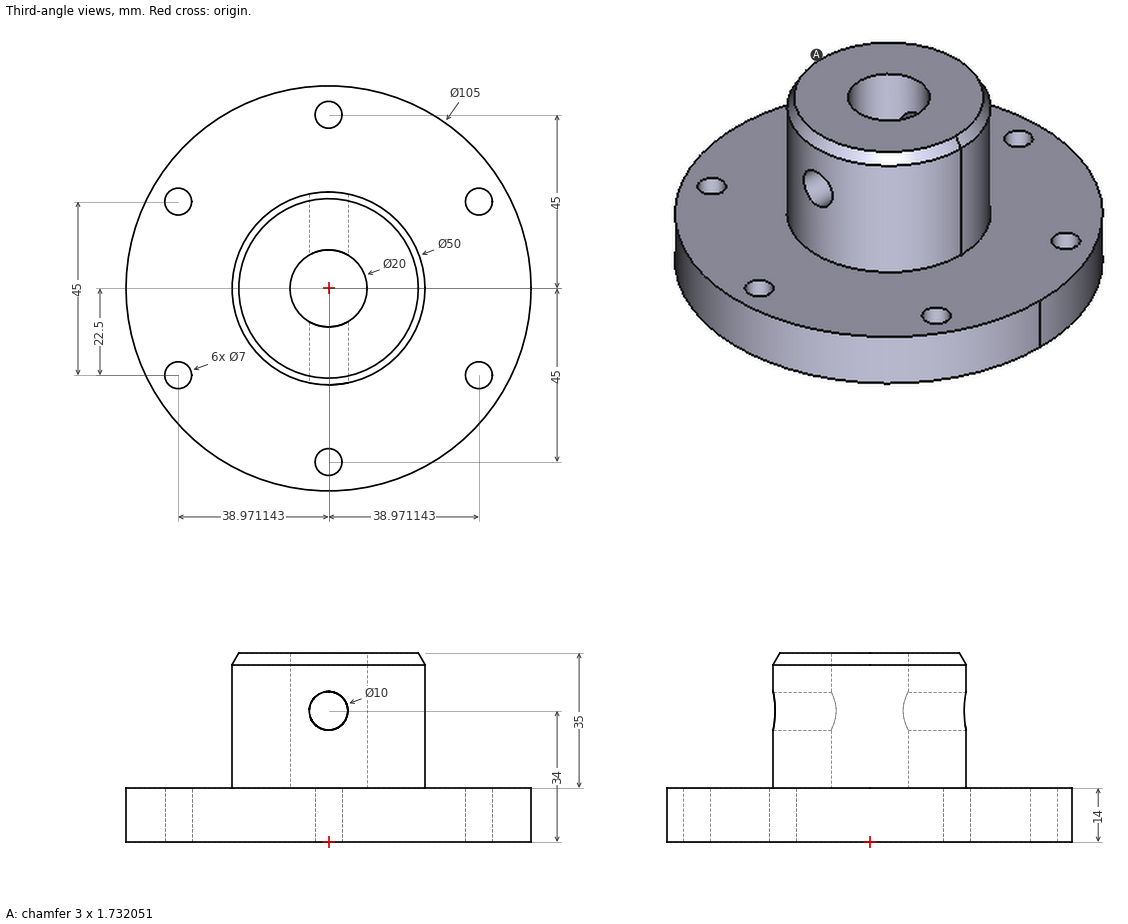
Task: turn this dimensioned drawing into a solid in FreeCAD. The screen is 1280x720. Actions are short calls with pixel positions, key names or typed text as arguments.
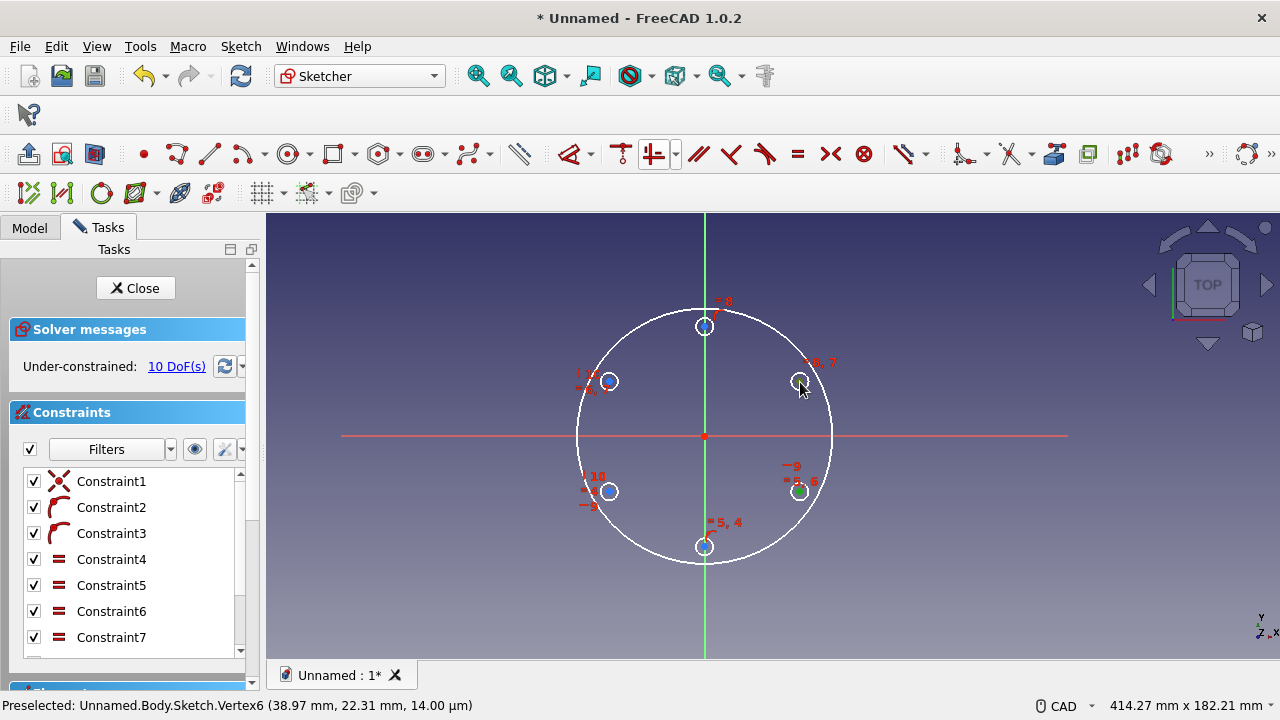
click(676, 154)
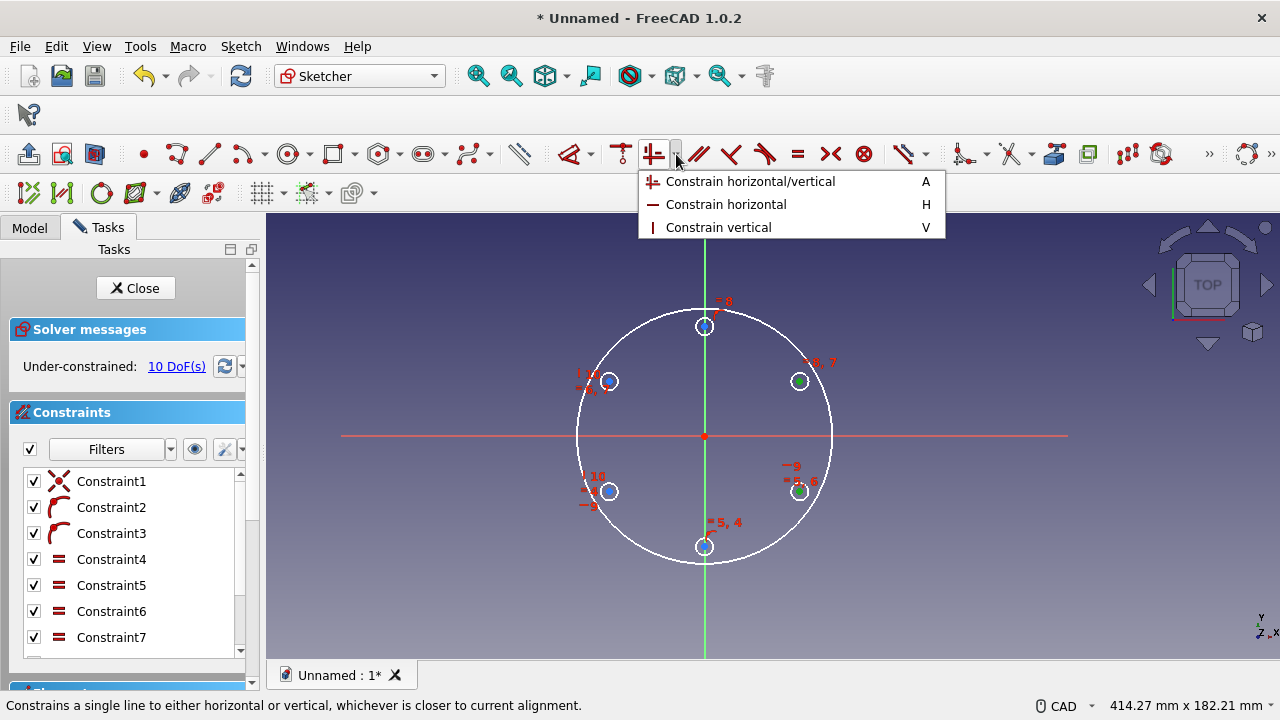
click(792, 228)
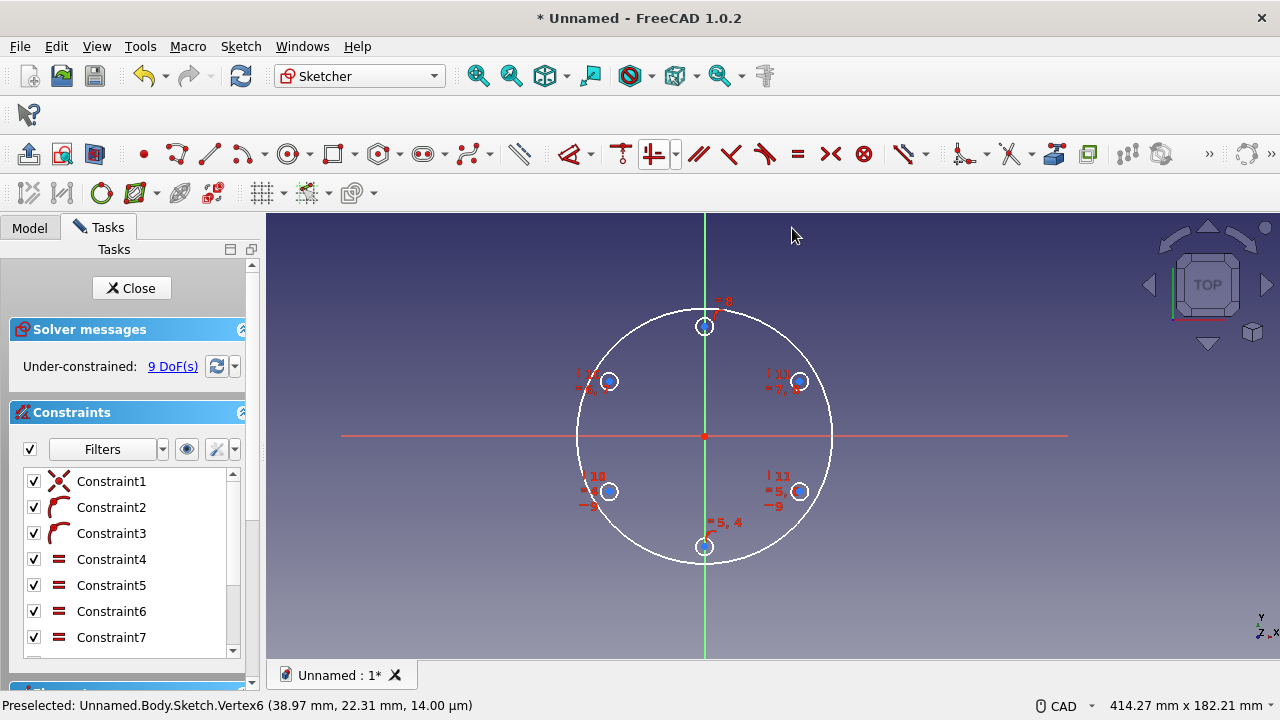
click(611, 384)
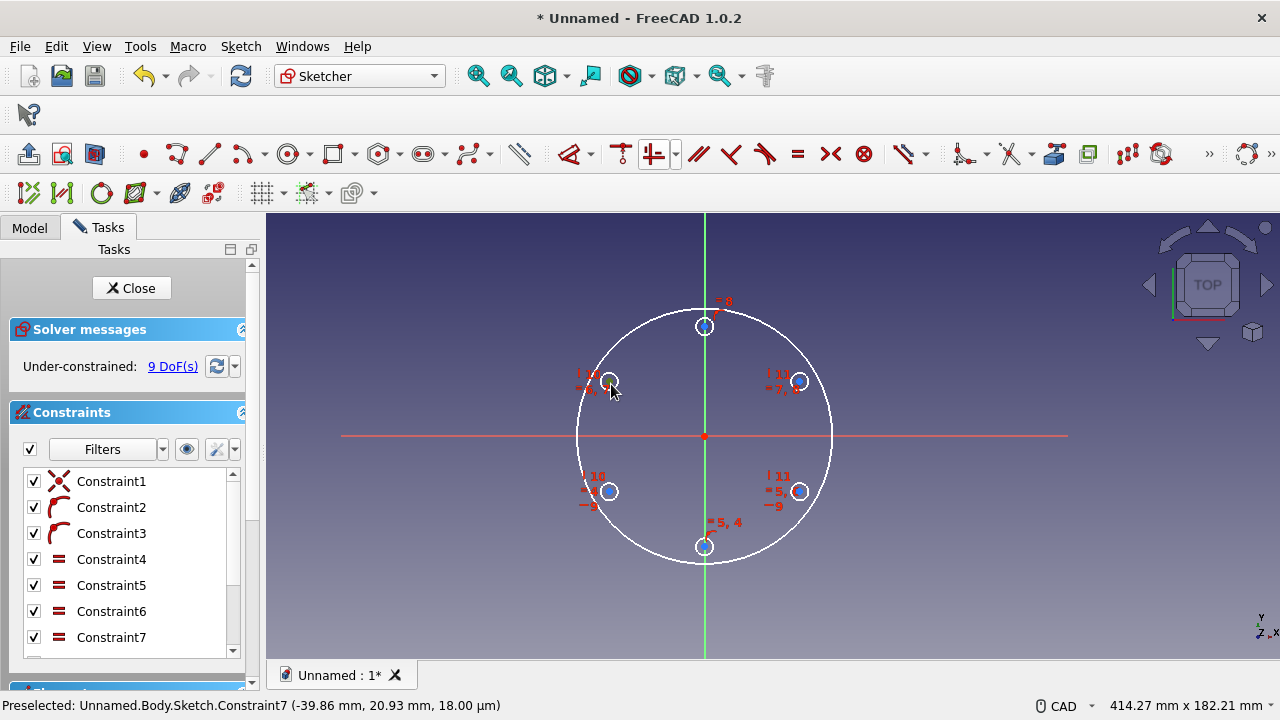
click(802, 384)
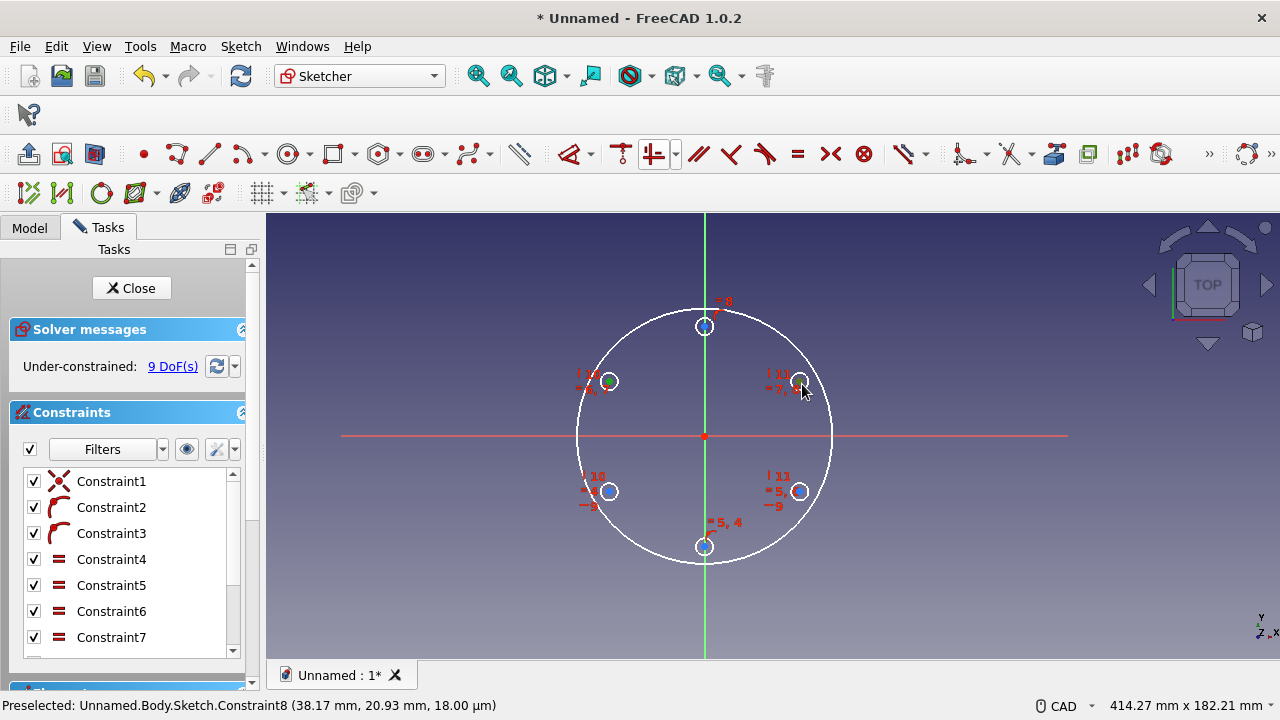
click(676, 154)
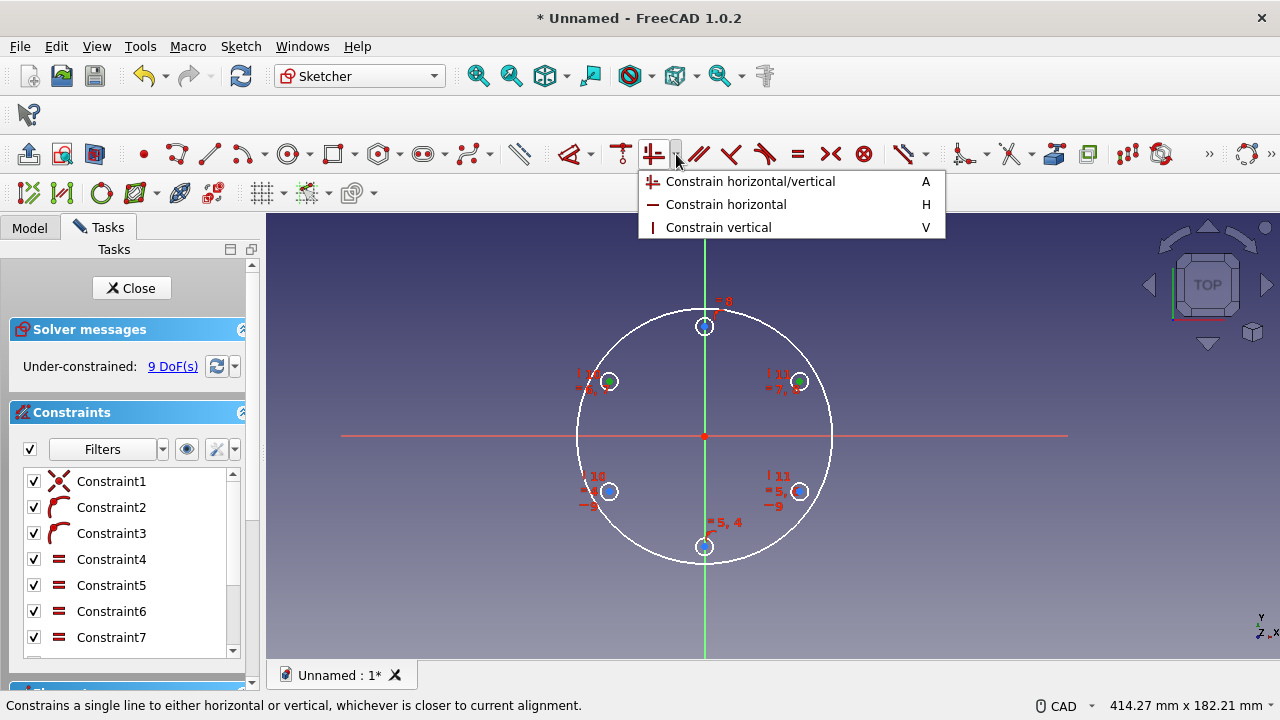
click(792, 204)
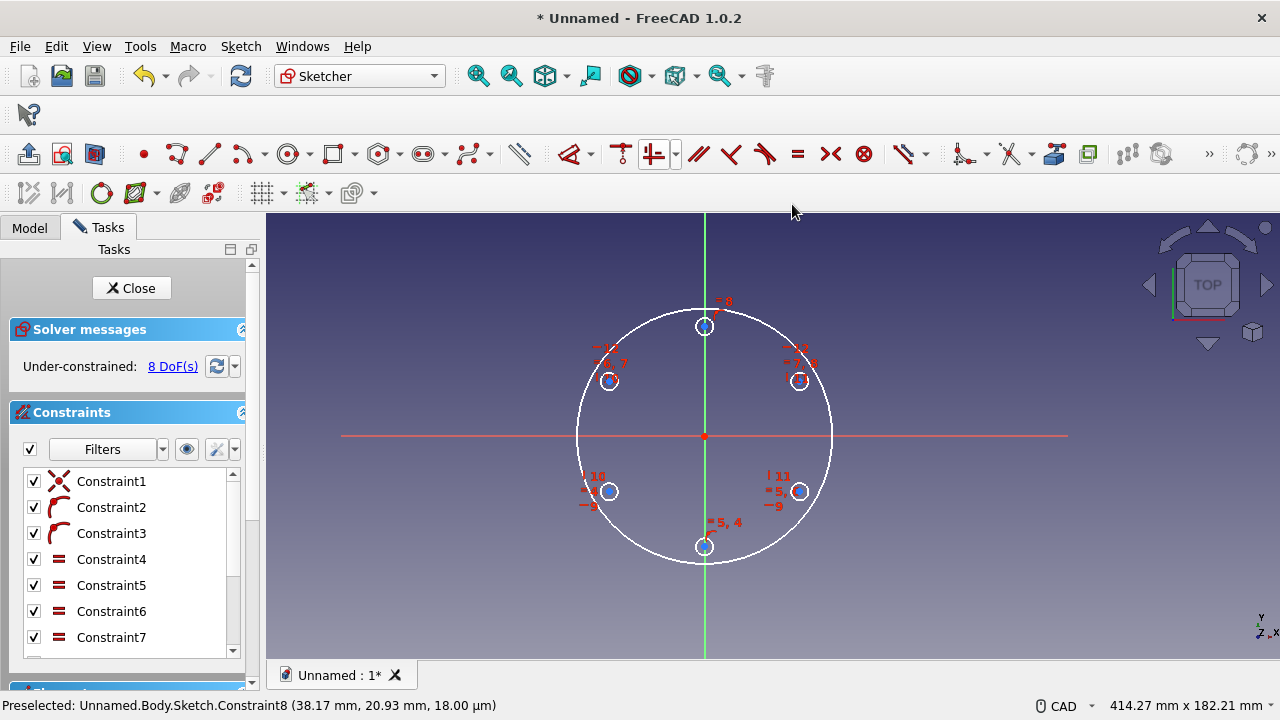
click(568, 154)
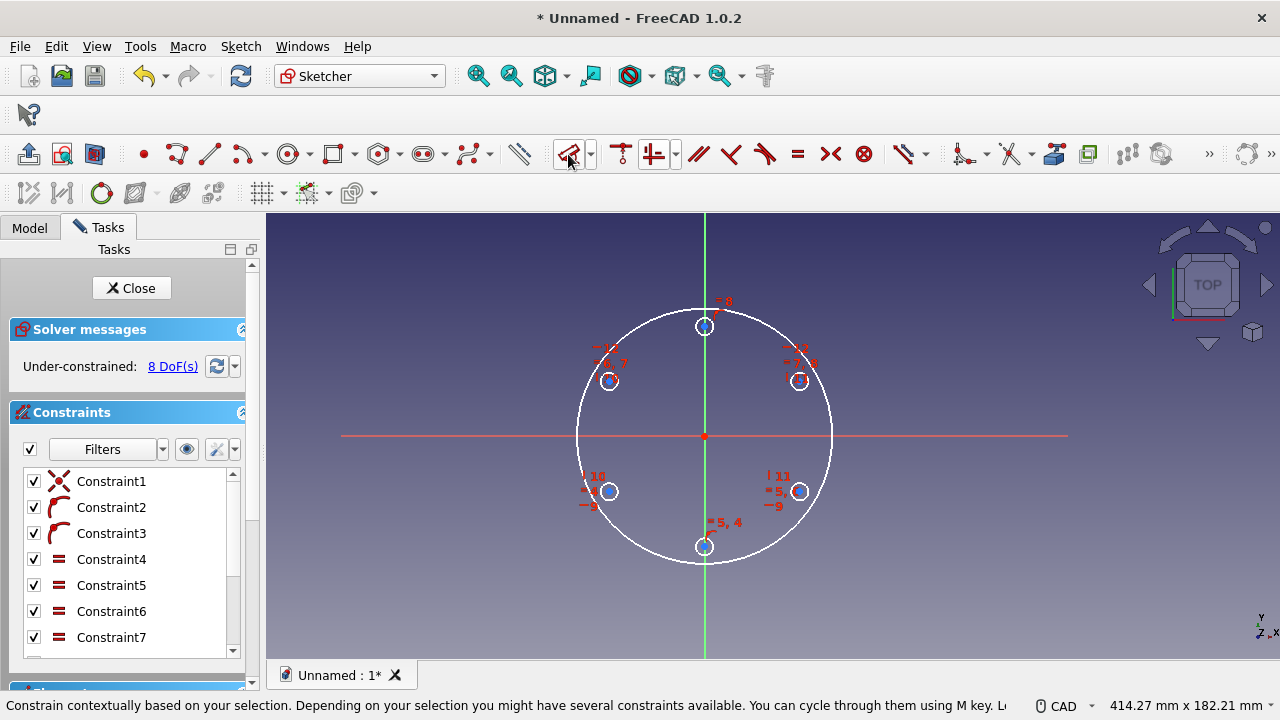
click(795, 346)
click(818, 323)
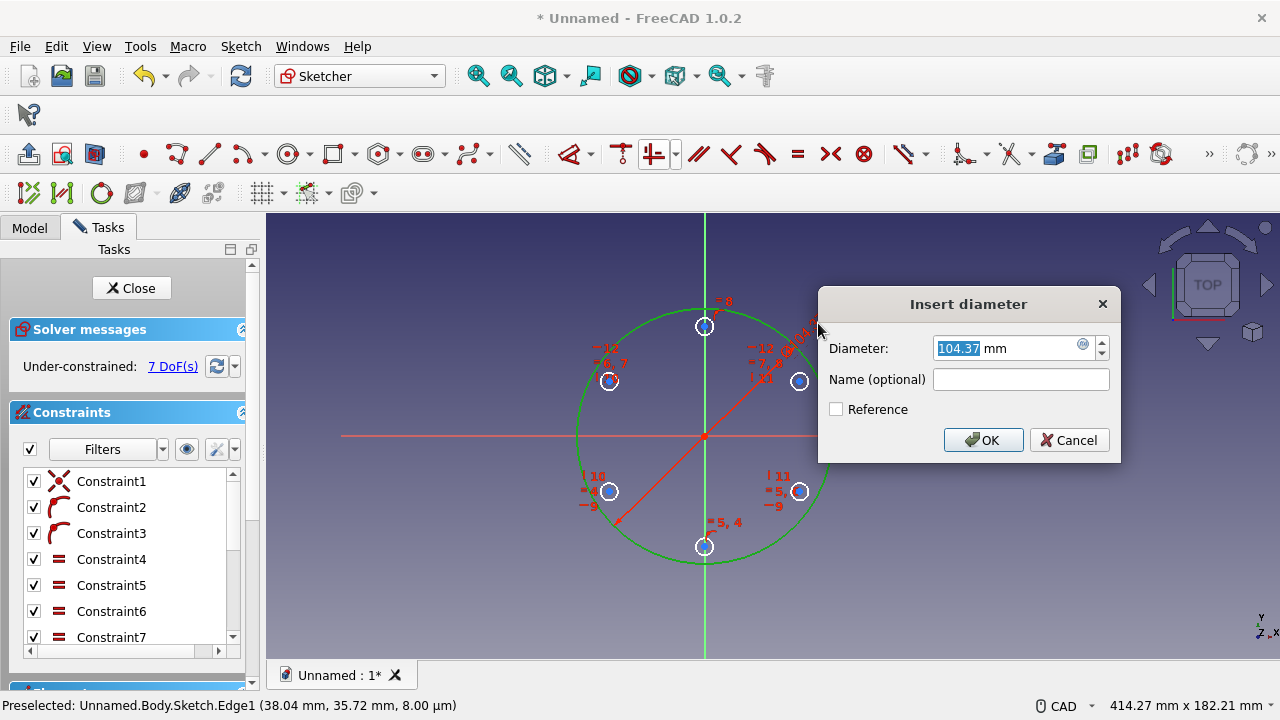
text(105)
key(Return)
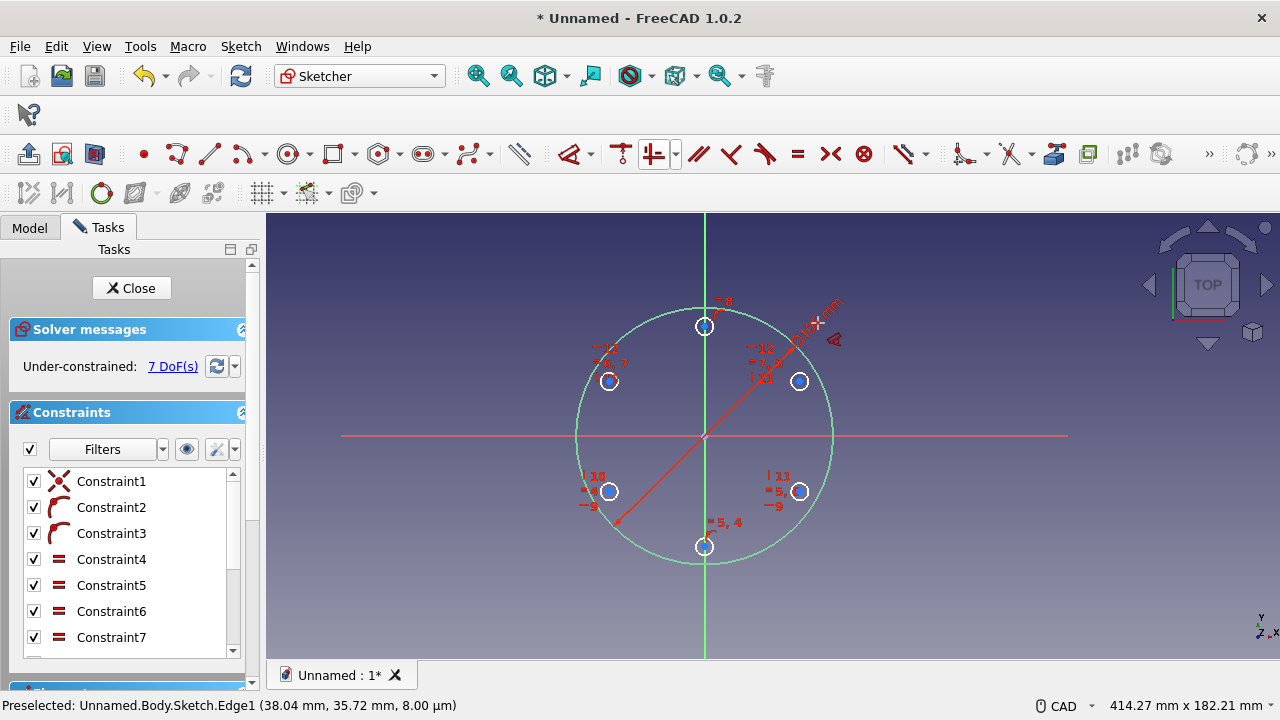
scroll(615, 486, up, 5)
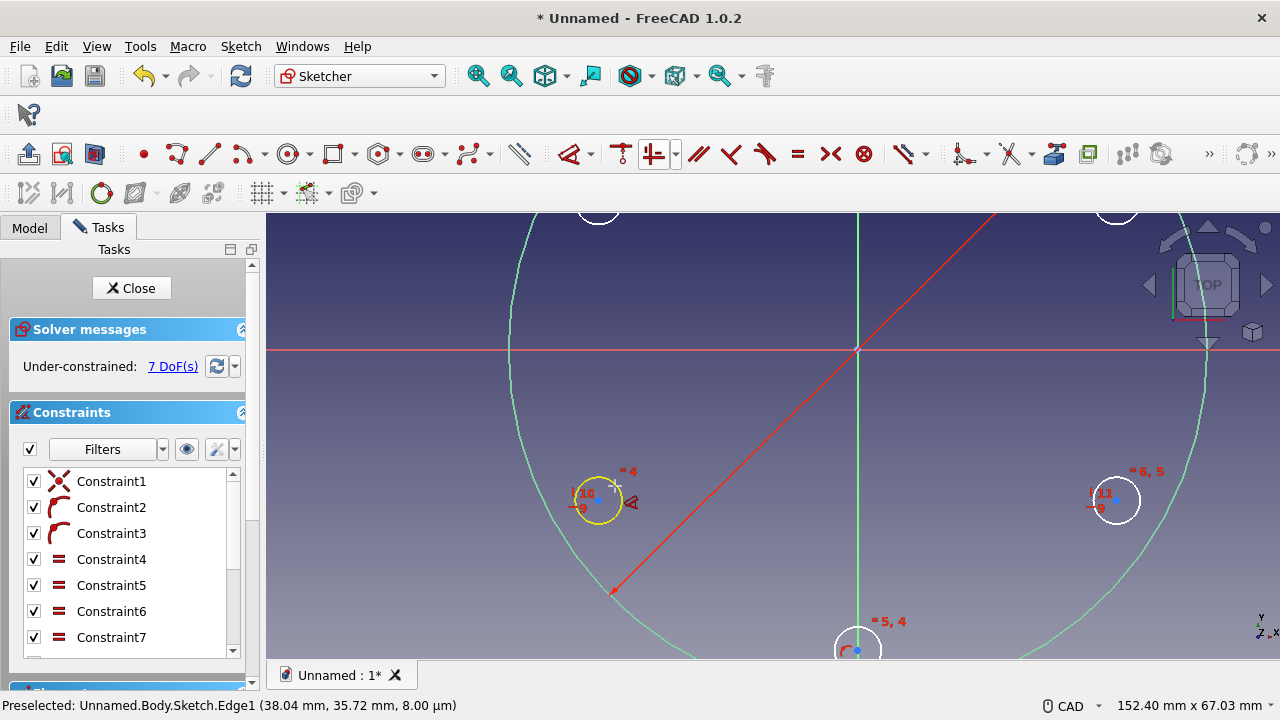
click(615, 484)
click(637, 461)